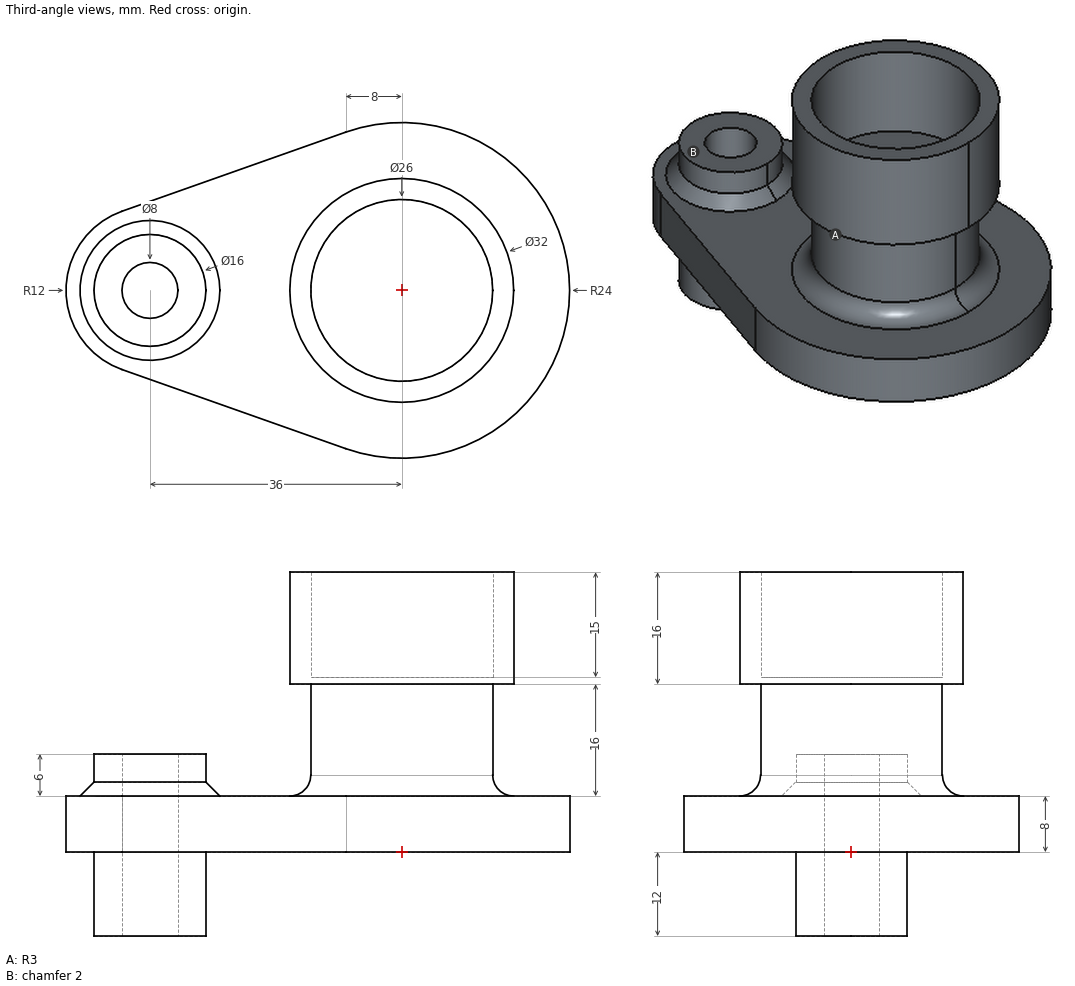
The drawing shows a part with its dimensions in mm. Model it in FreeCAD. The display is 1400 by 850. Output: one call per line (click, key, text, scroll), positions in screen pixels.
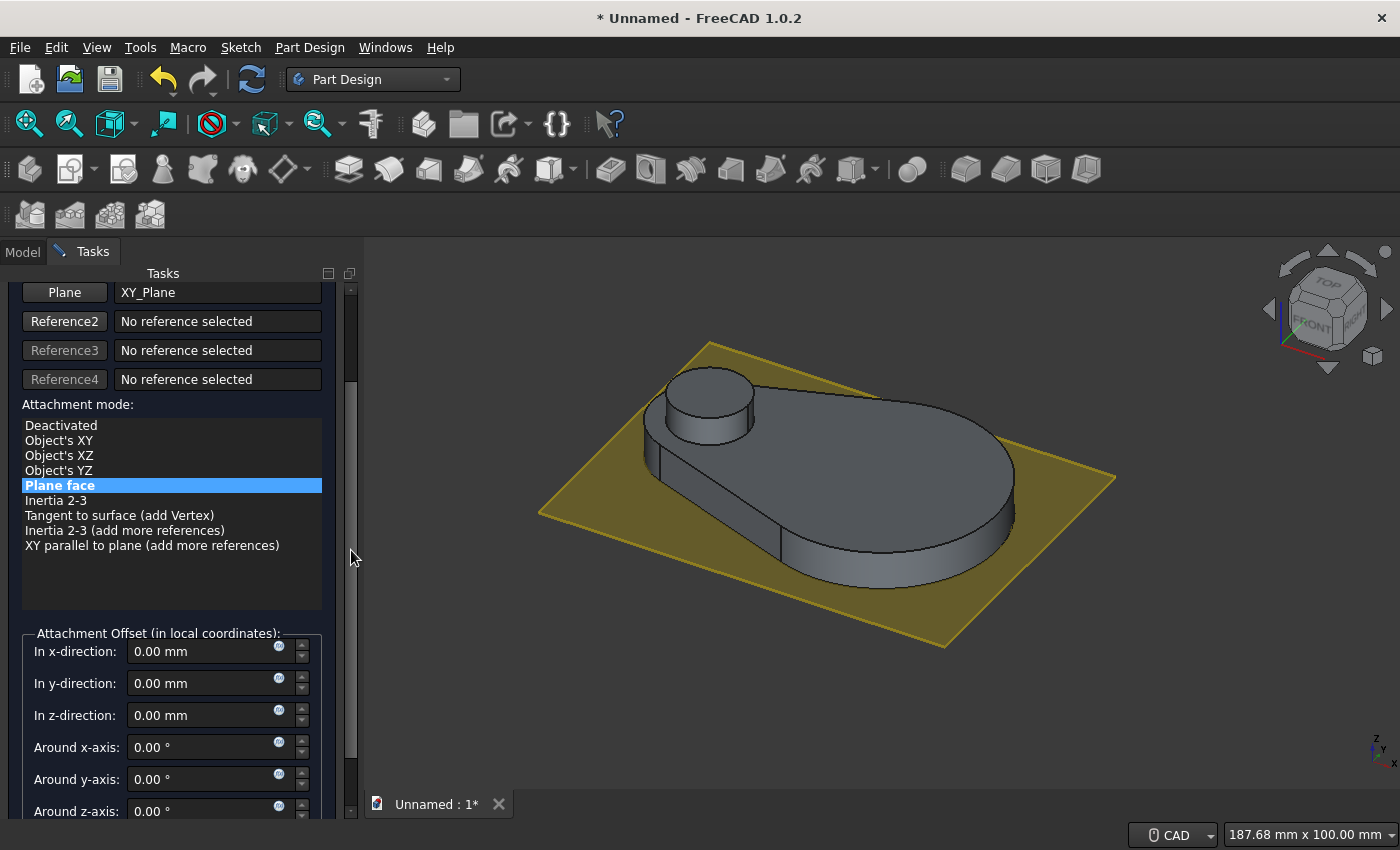
triple_click(210, 715)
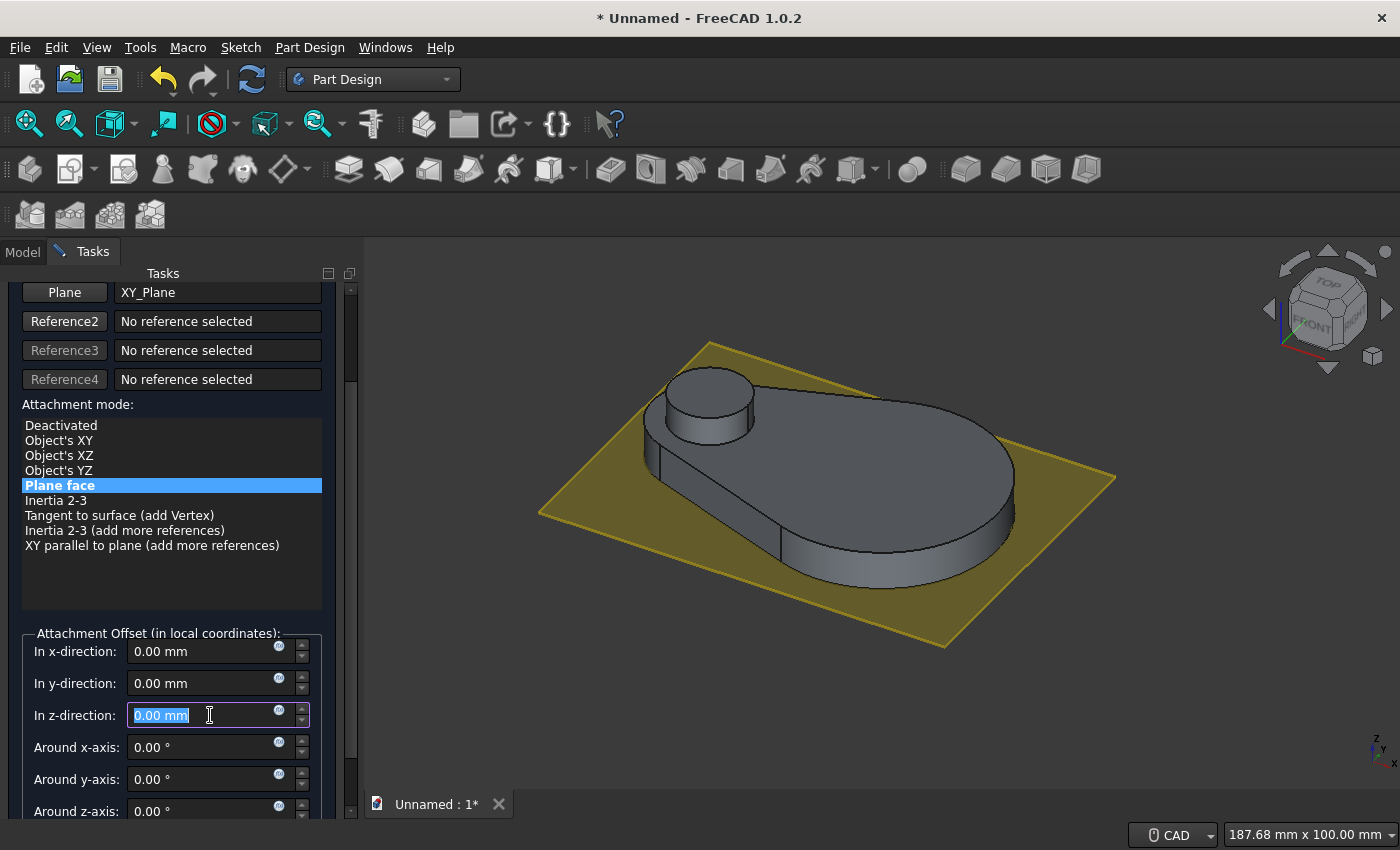
text(-12)
key(Tab)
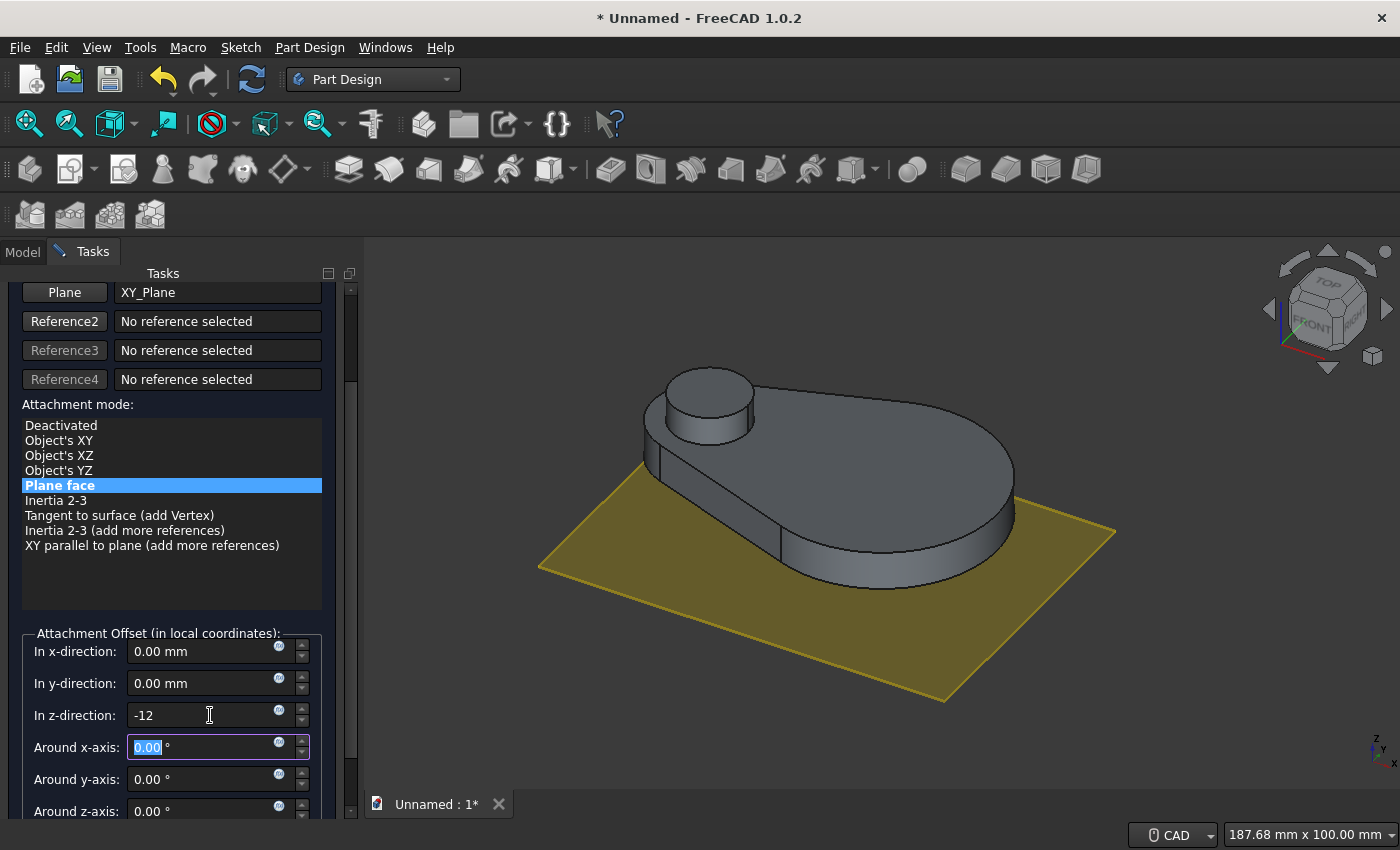
scroll(351, 550, up, 3)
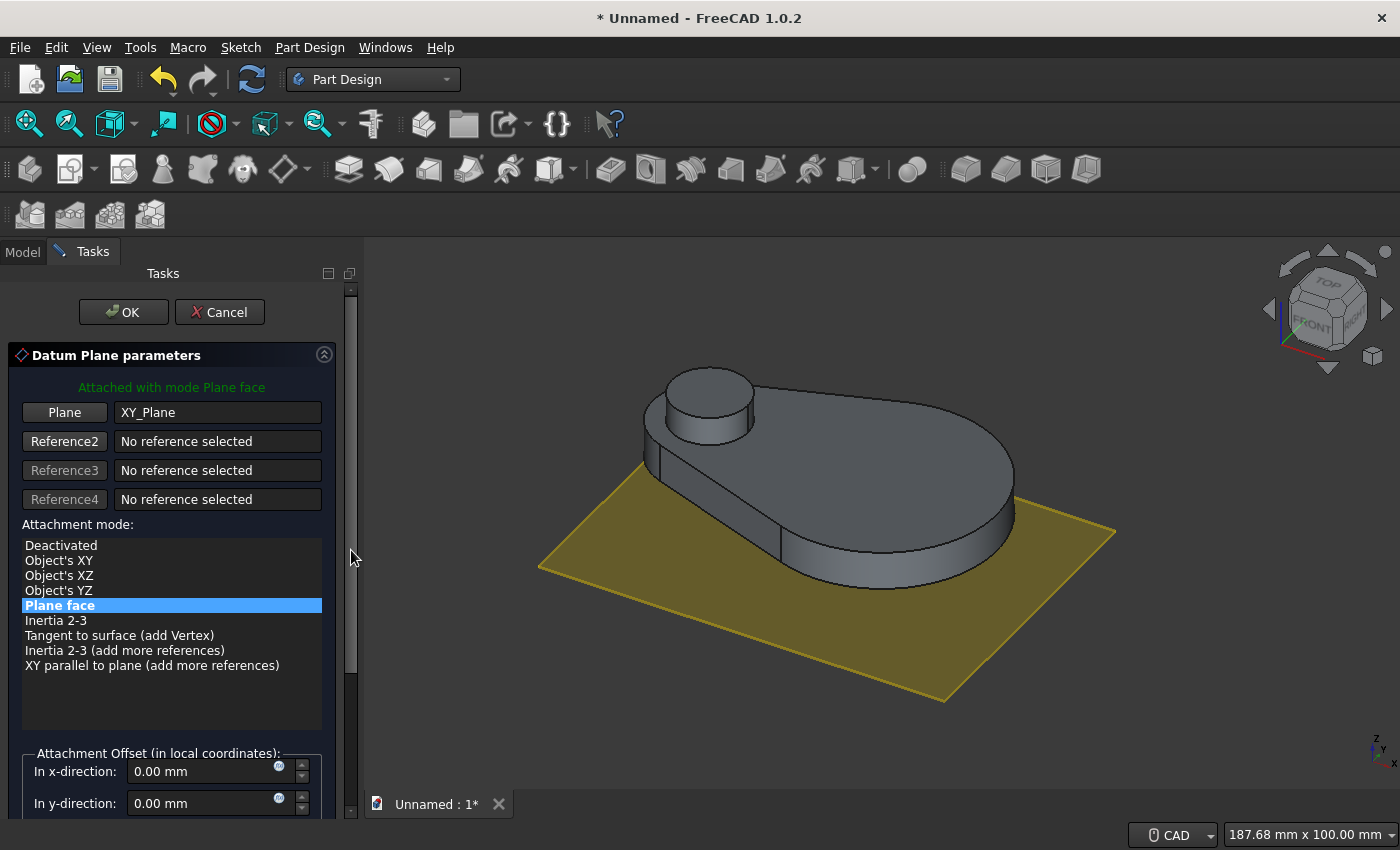
click(124, 312)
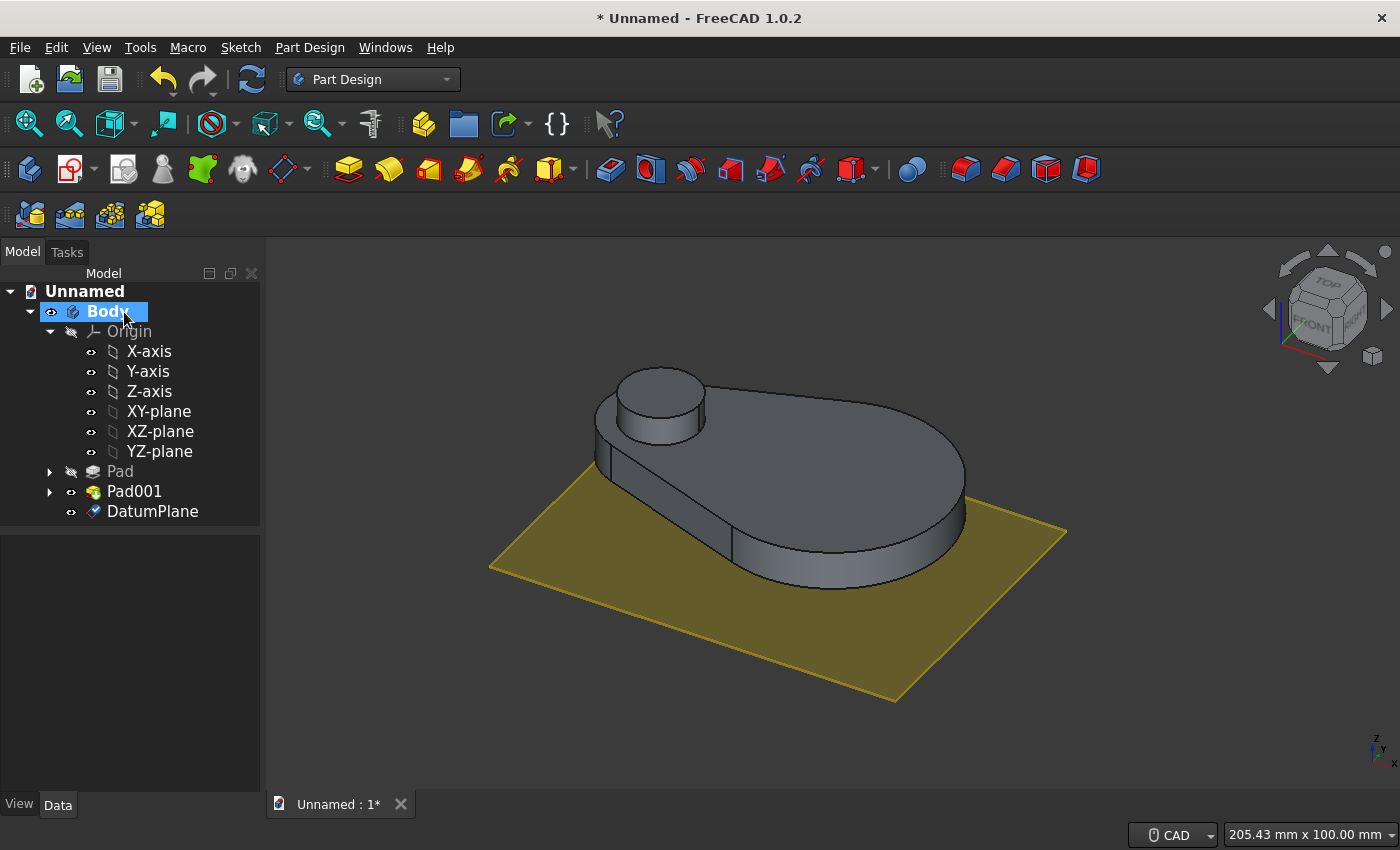
click(116, 512)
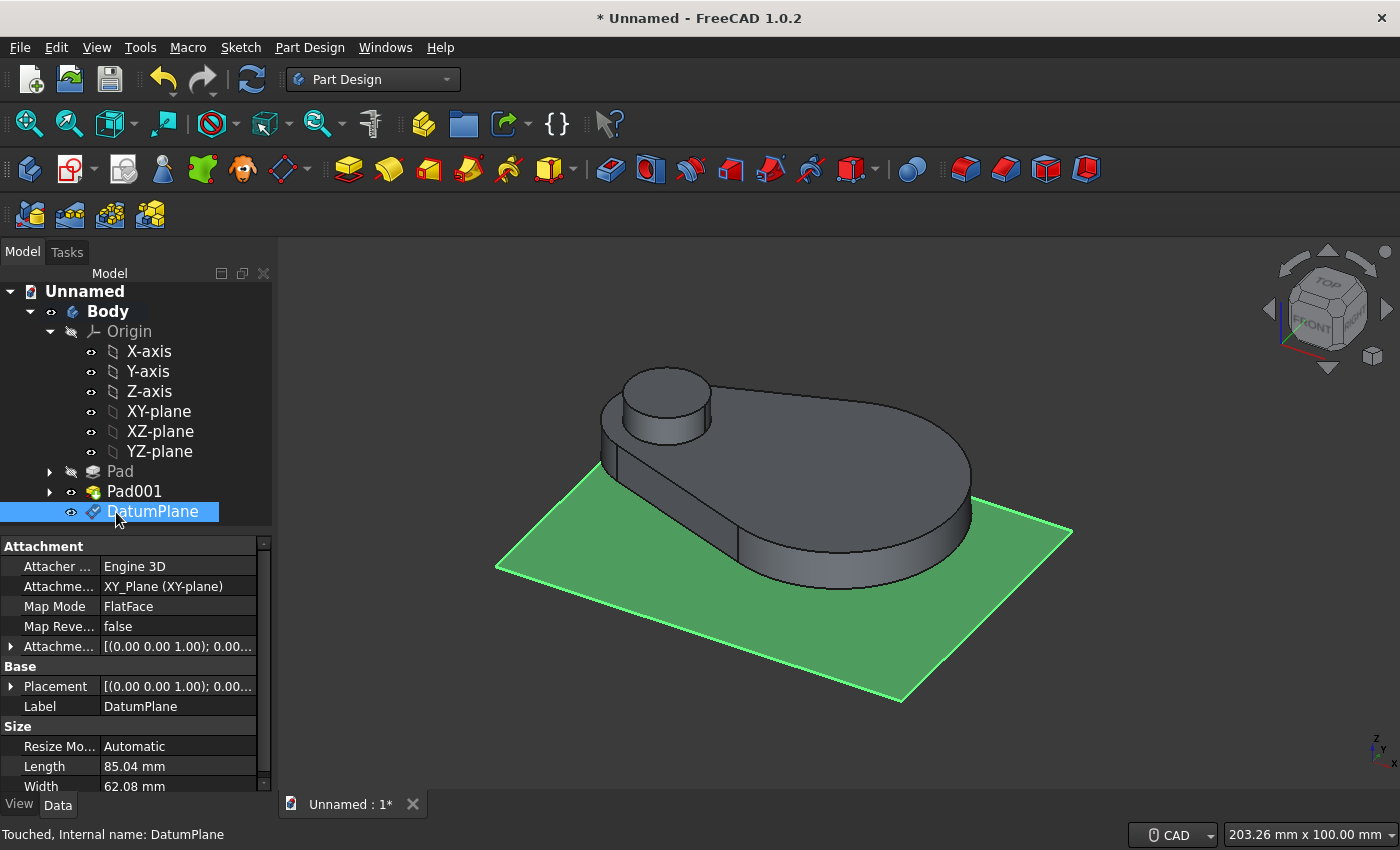
click(70, 170)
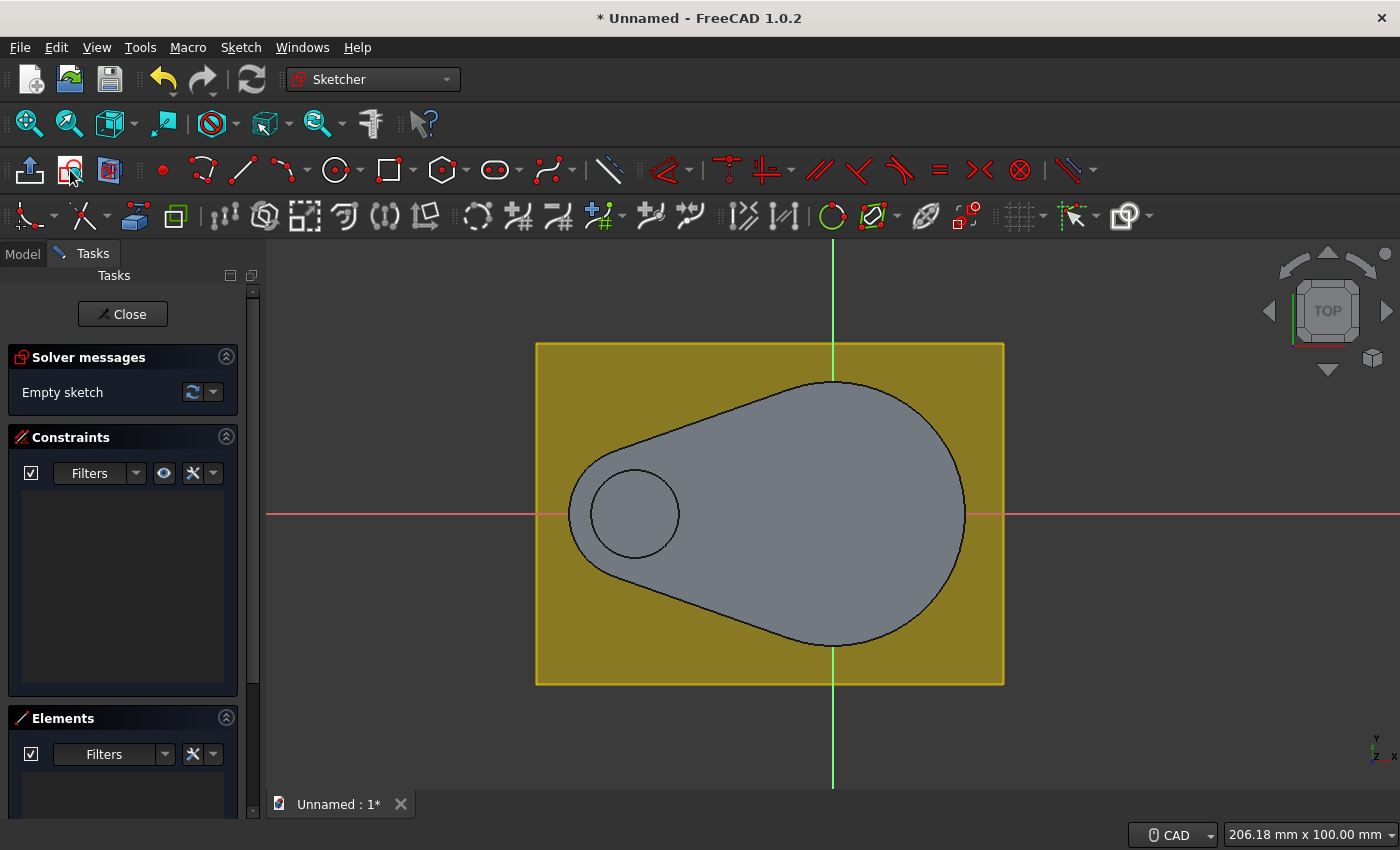
click(110, 170)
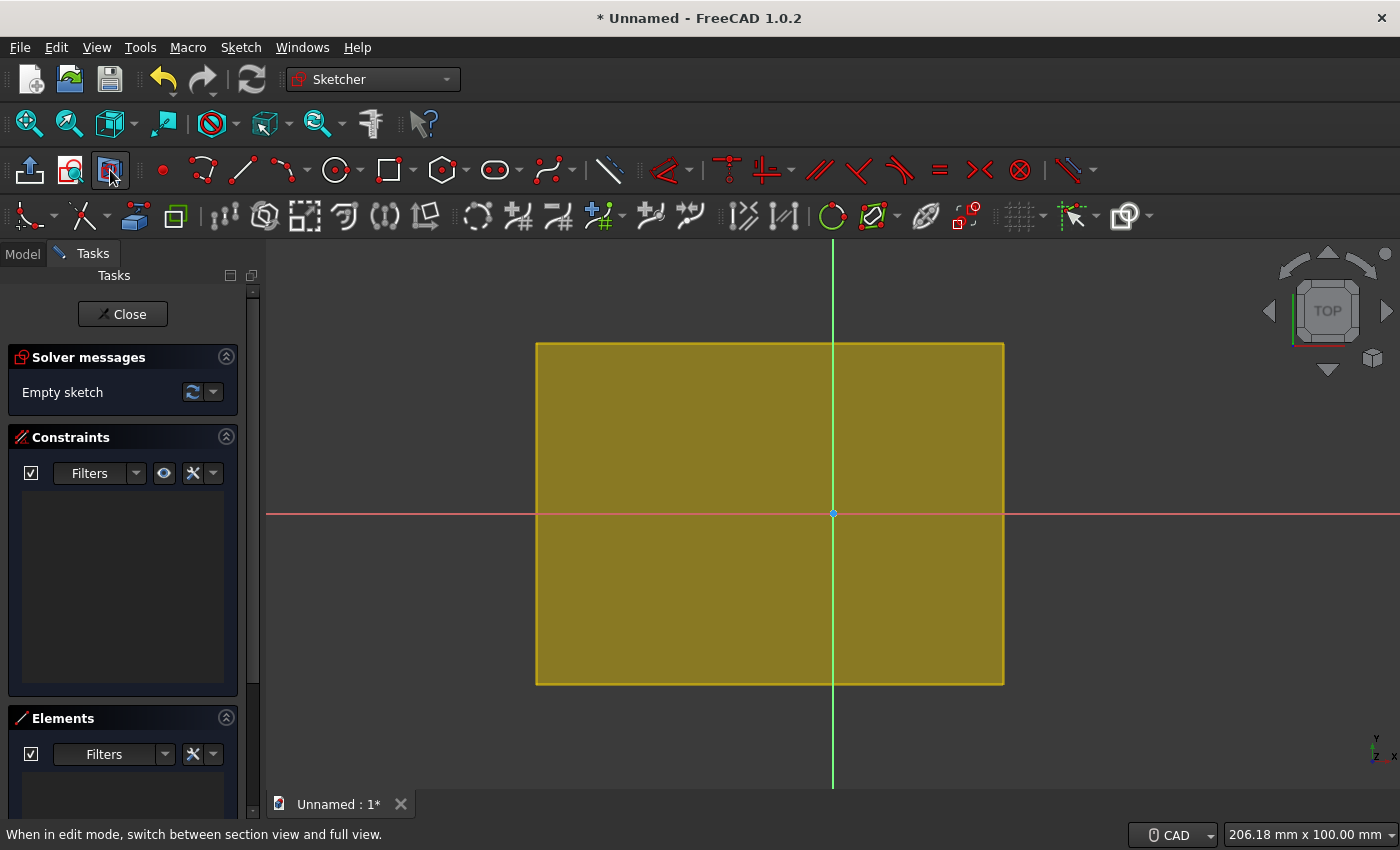
scroll(593, 514, up, 7)